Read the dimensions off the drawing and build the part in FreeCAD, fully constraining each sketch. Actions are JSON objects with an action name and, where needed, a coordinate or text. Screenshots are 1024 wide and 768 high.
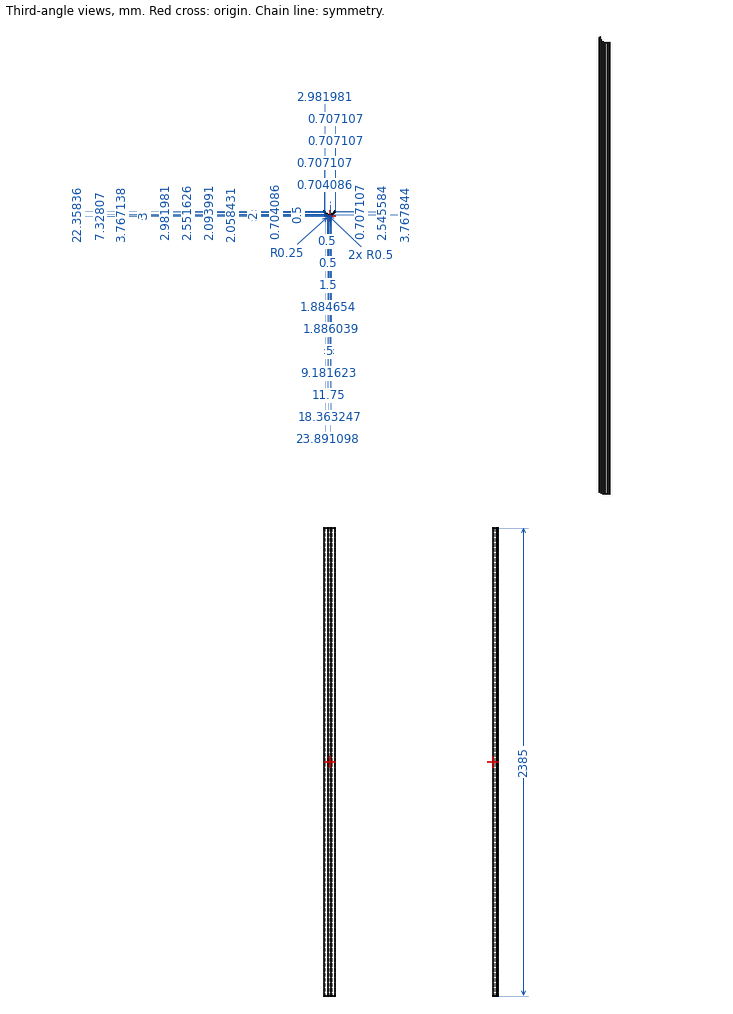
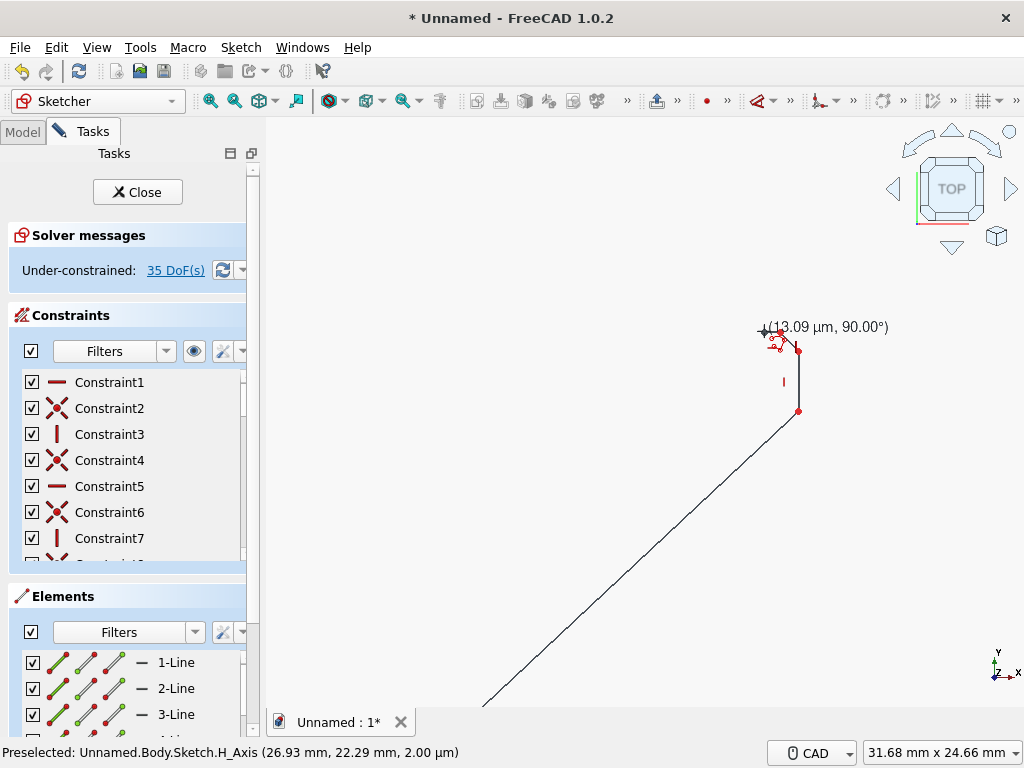
{"action": "scroll", "coordinate": [773, 331], "scroll_direction": "down", "scroll_amount": 6}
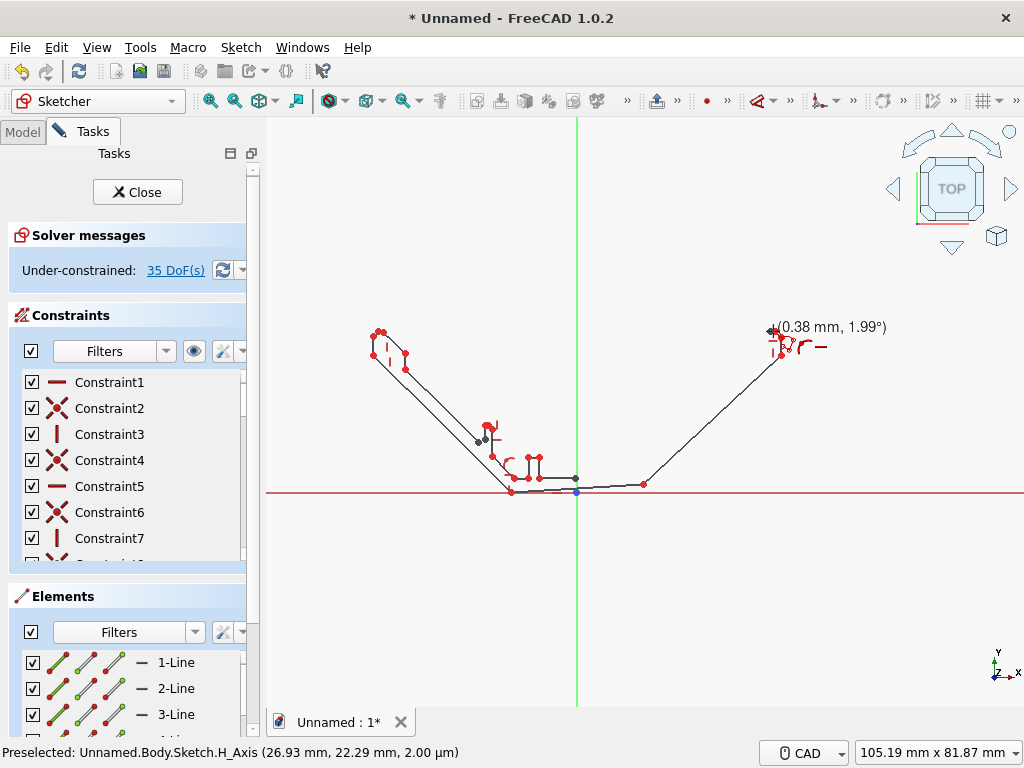
{"action": "left_click", "coordinate": [749, 353]}
{"action": "left_click", "coordinate": [749, 368]}
{"action": "left_click", "coordinate": [675, 442]}
{"action": "right_click", "coordinate": [675, 442]}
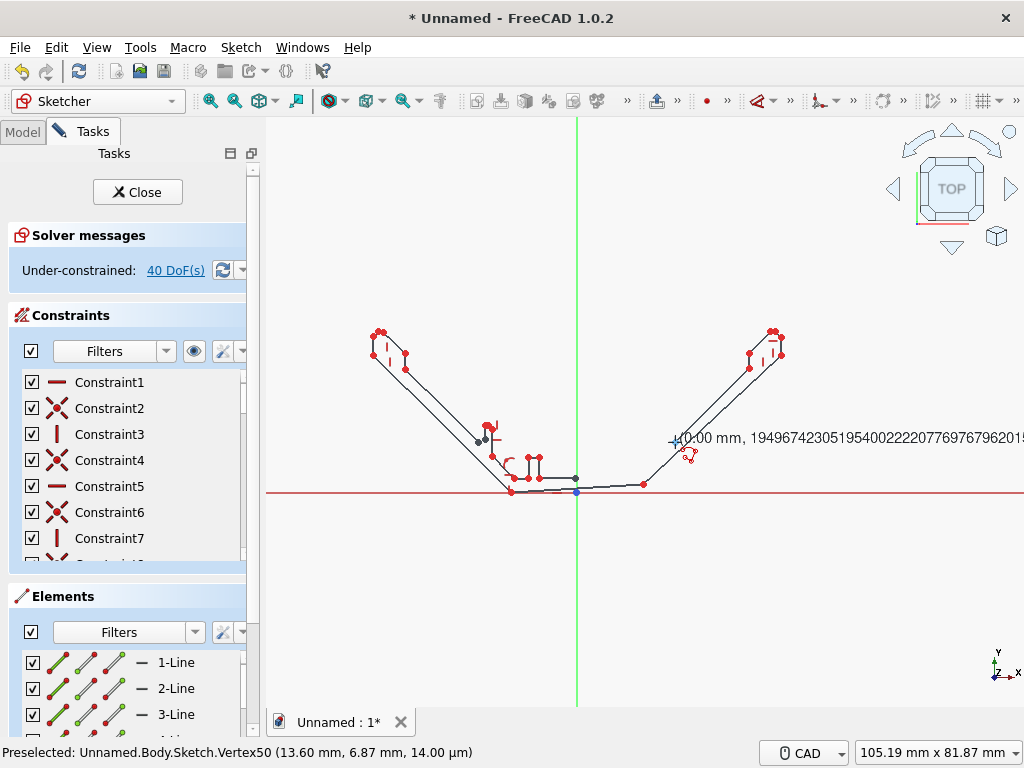
{"action": "scroll", "coordinate": [669, 440], "scroll_direction": "up", "scroll_amount": 5}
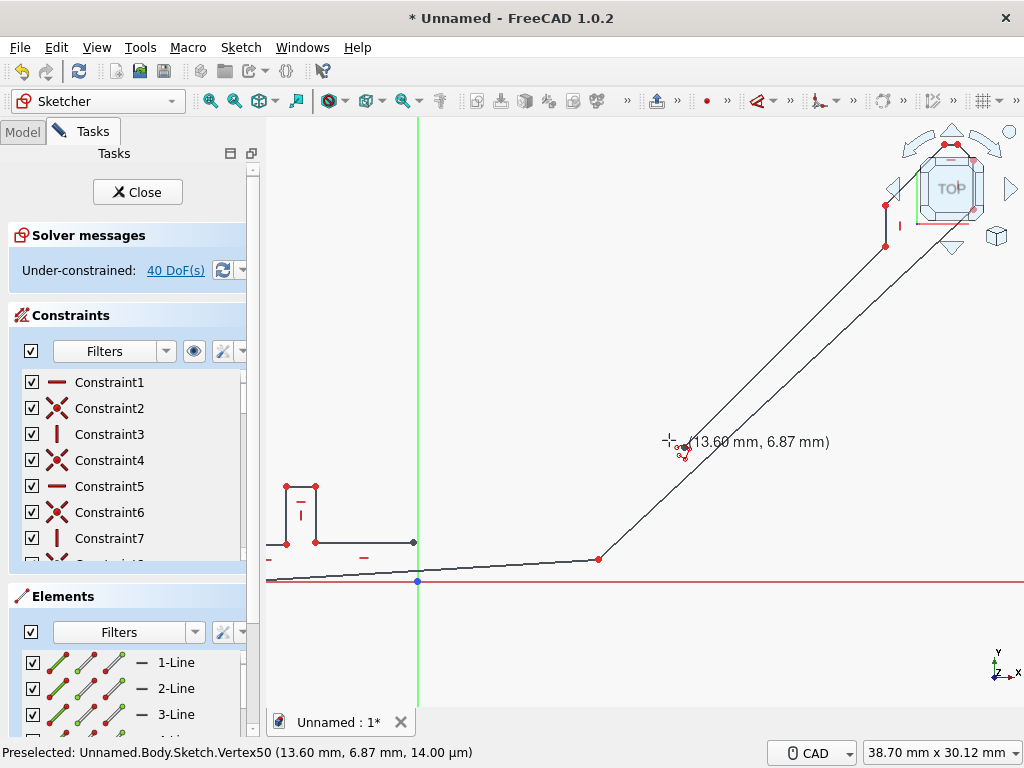
{"action": "left_click", "coordinate": [668, 438]}
{"action": "left_click", "coordinate": [668, 398]}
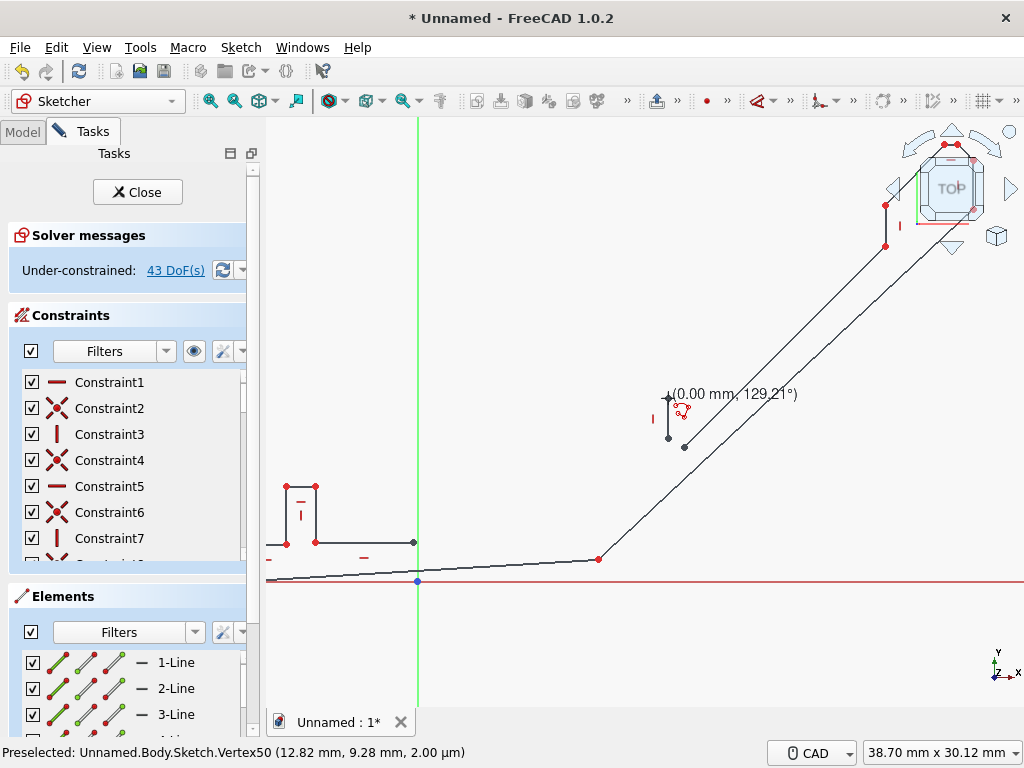
{"action": "scroll", "coordinate": [658, 398], "scroll_direction": "up", "scroll_amount": 3}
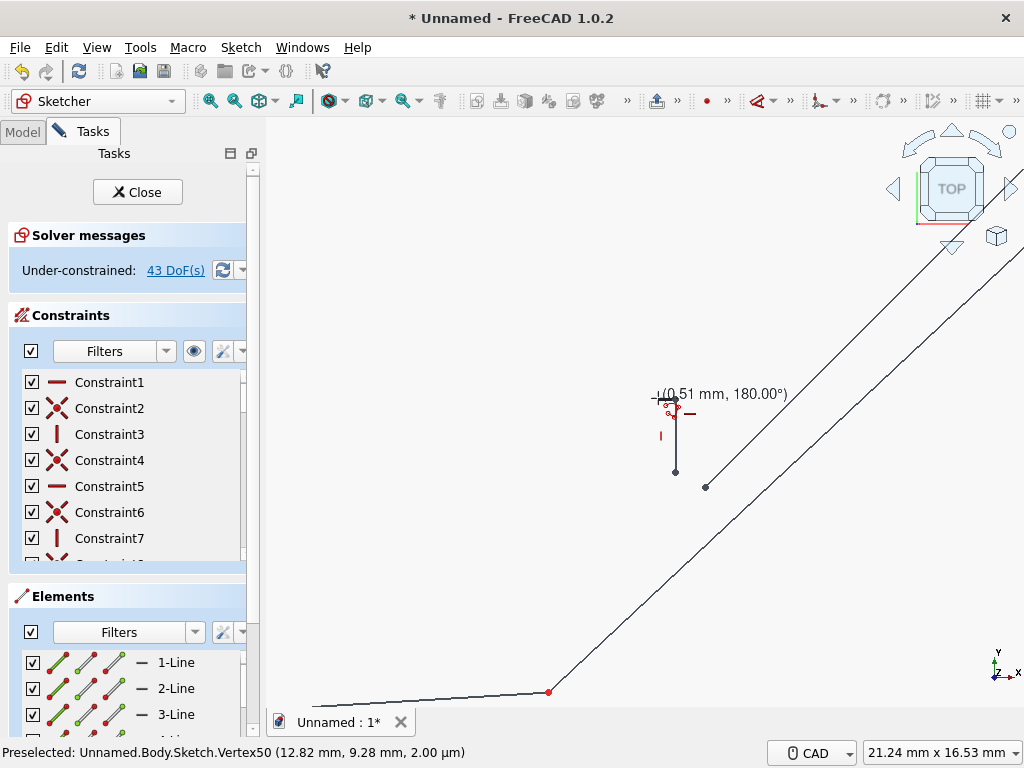
{"action": "left_click", "coordinate": [657, 398]}
{"action": "left_click", "coordinate": [640, 415]}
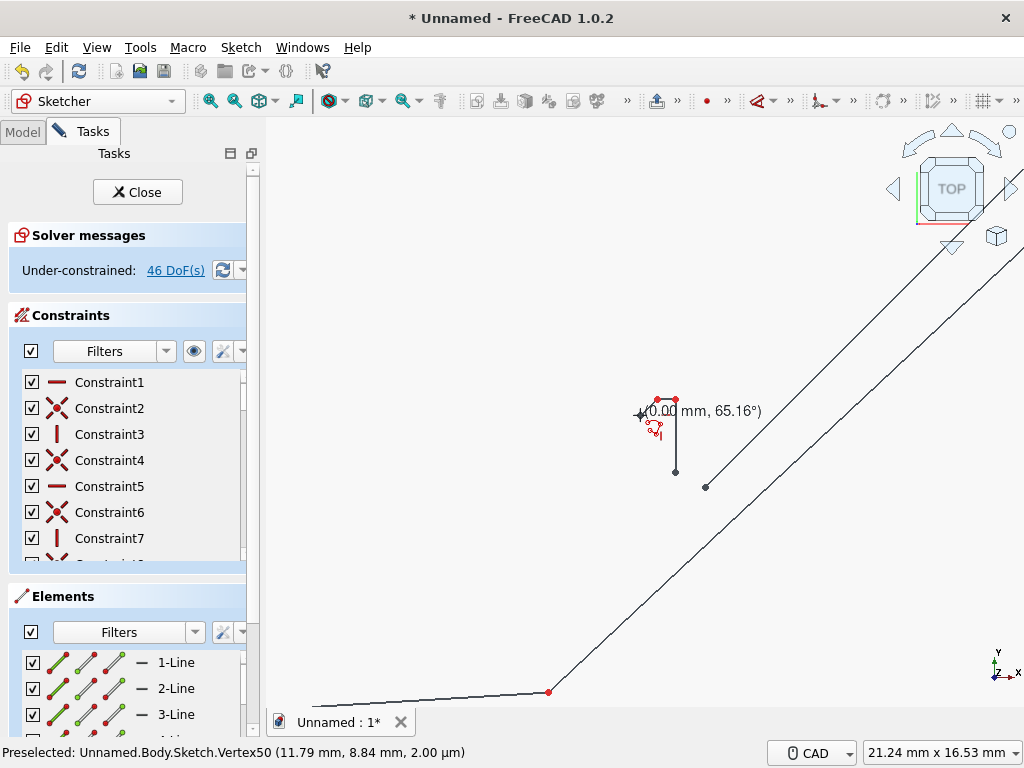
{"action": "scroll", "coordinate": [667, 432], "scroll_direction": "down", "scroll_amount": 8}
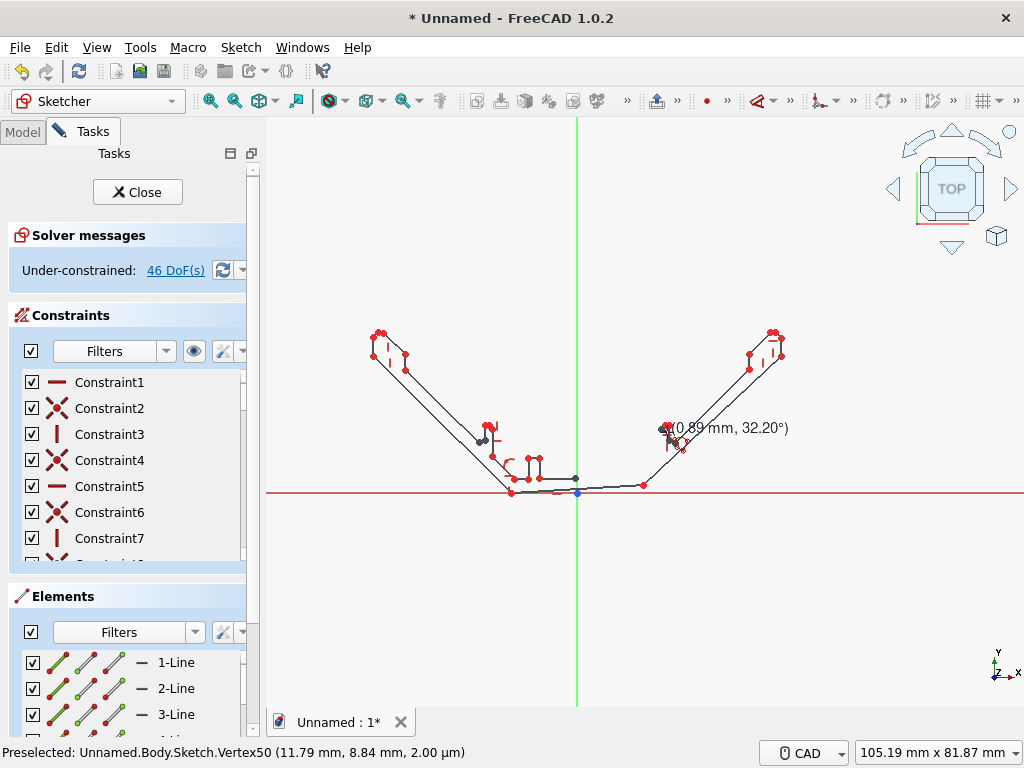
{"action": "scroll", "coordinate": [662, 456], "scroll_direction": "up", "scroll_amount": 2}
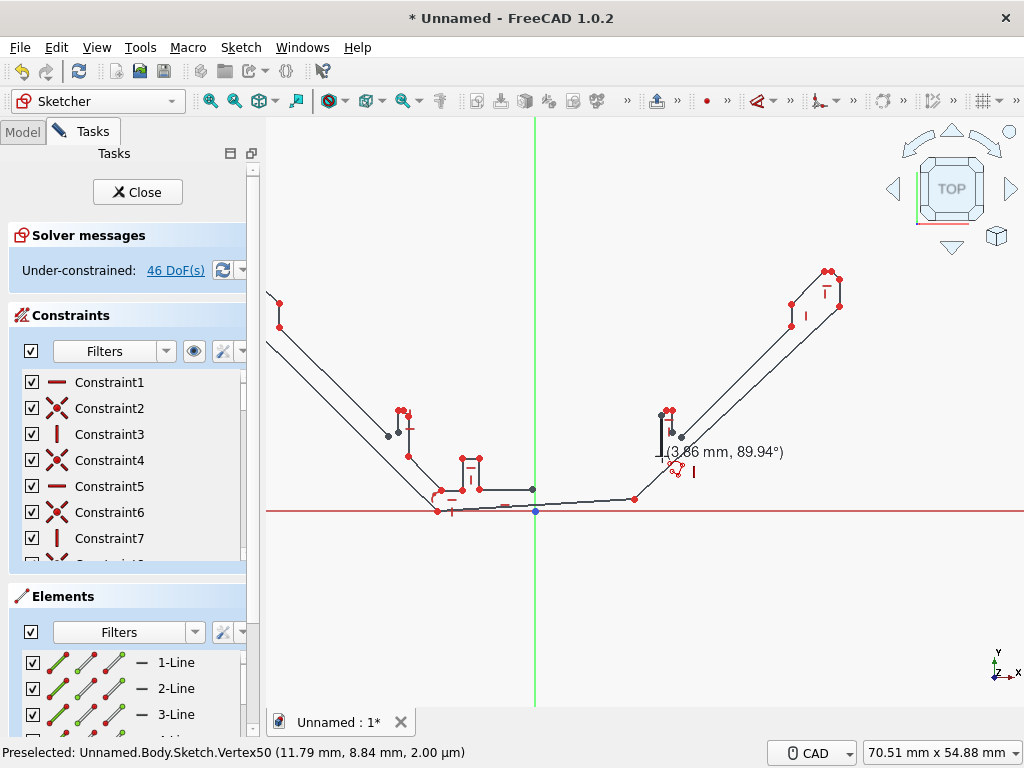
{"action": "left_click", "coordinate": [662, 456]}
{"action": "left_click", "coordinate": [628, 490]}
{"action": "left_click", "coordinate": [608, 490]}
{"action": "left_click", "coordinate": [608, 457]}
{"action": "left_click", "coordinate": [592, 457]}
{"action": "left_click", "coordinate": [592, 490]}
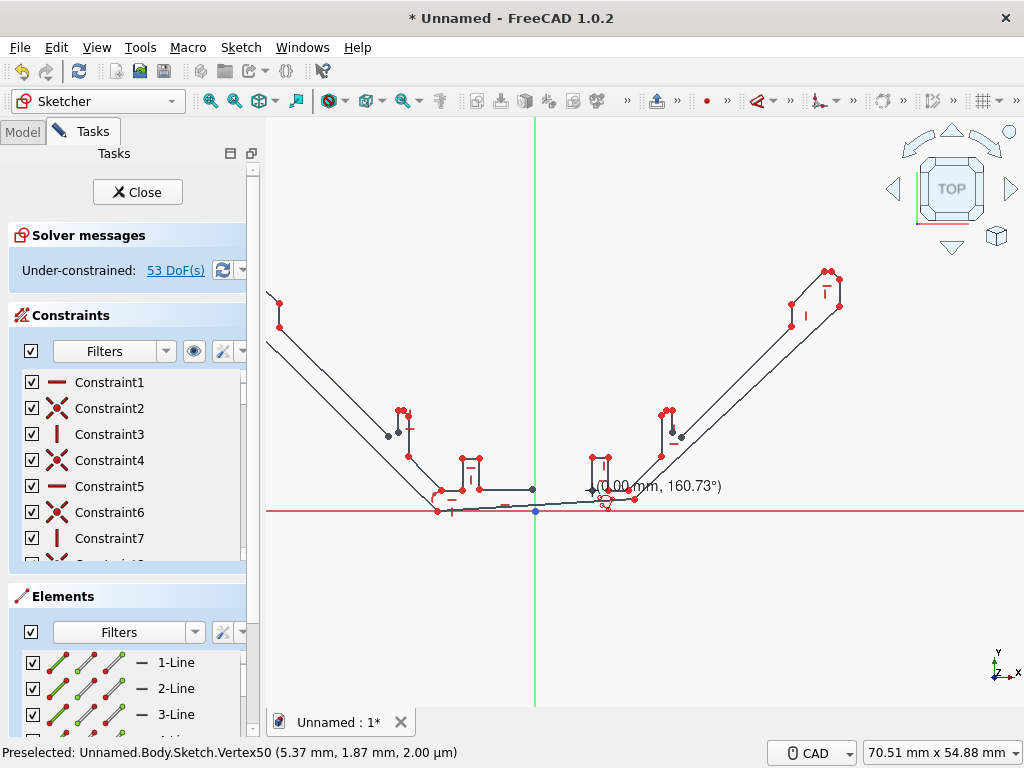
{"action": "scroll", "coordinate": [538, 490], "scroll_direction": "up", "scroll_amount": 9}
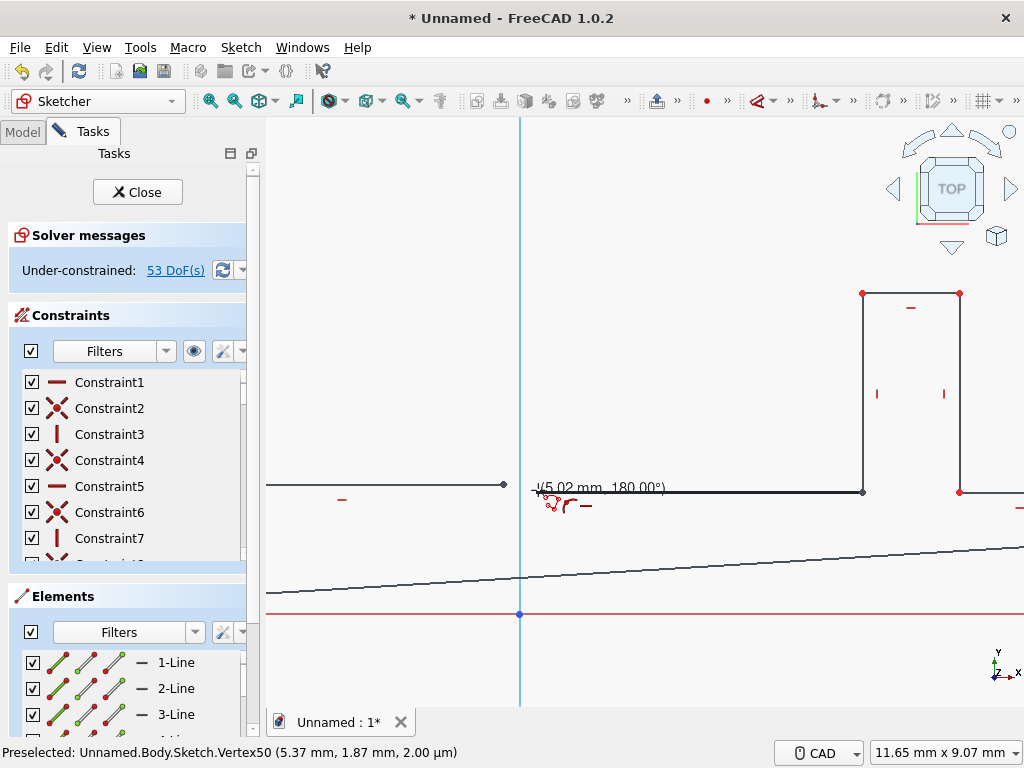
{"action": "left_click", "coordinate": [536, 487]}
{"action": "right_click", "coordinate": [536, 487]}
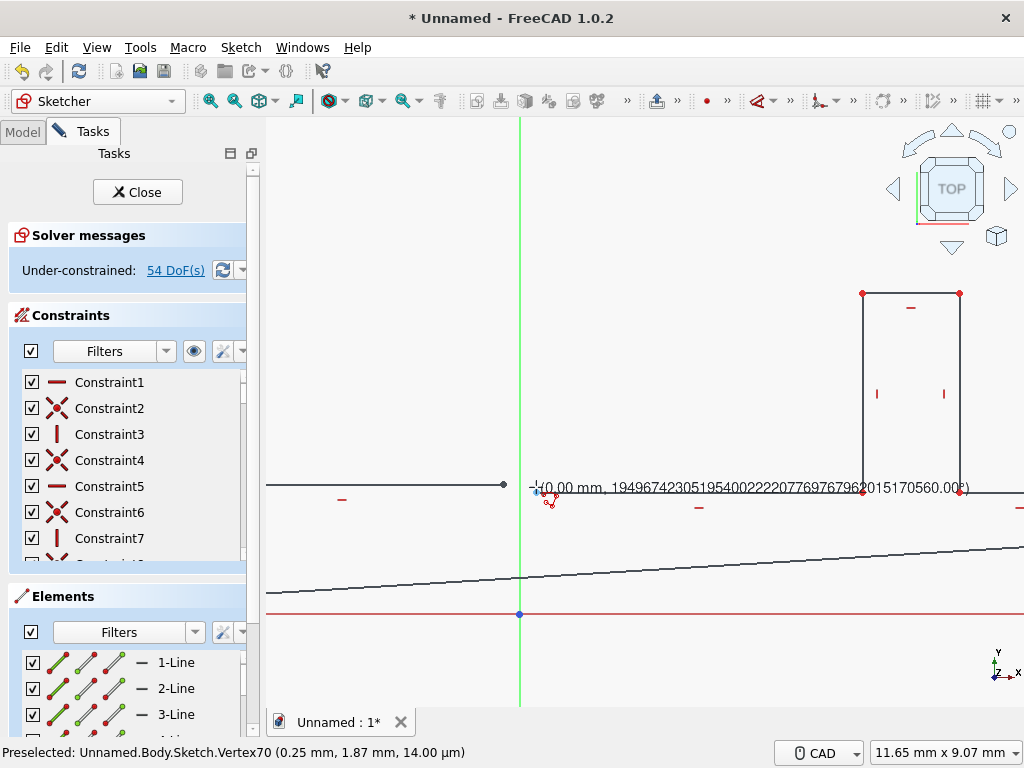
{"action": "key", "text": "g 3 a"}